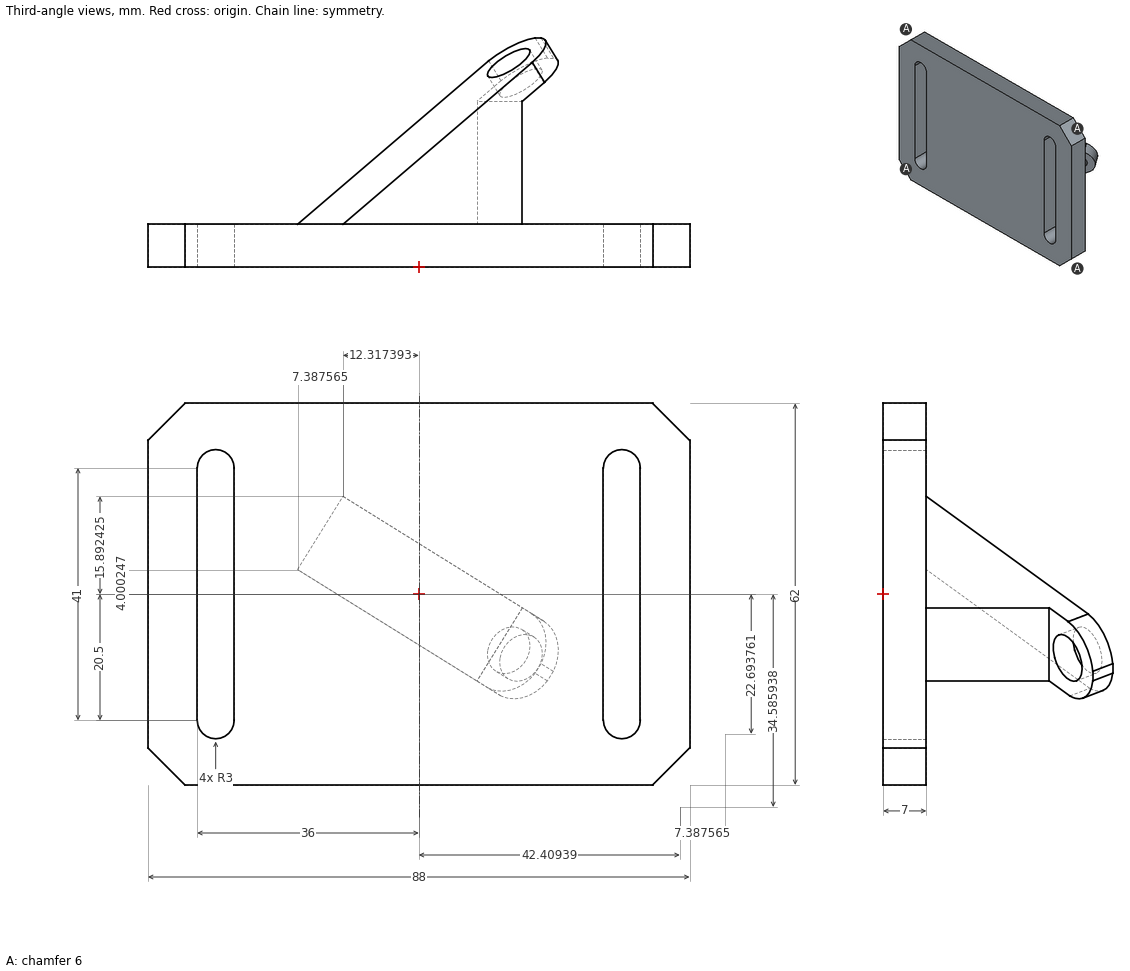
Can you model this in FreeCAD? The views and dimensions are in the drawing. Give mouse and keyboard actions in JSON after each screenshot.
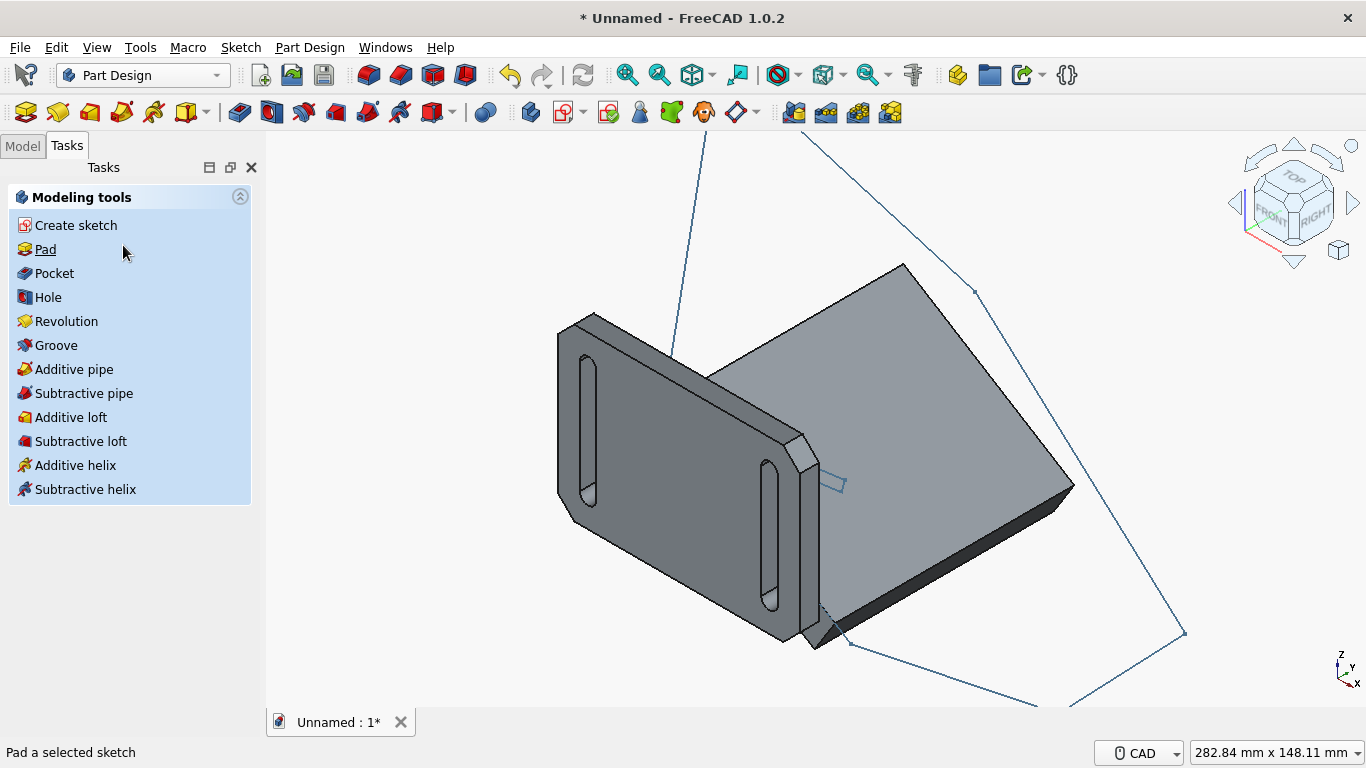
{"action": "left_click", "coordinate": [240, 112]}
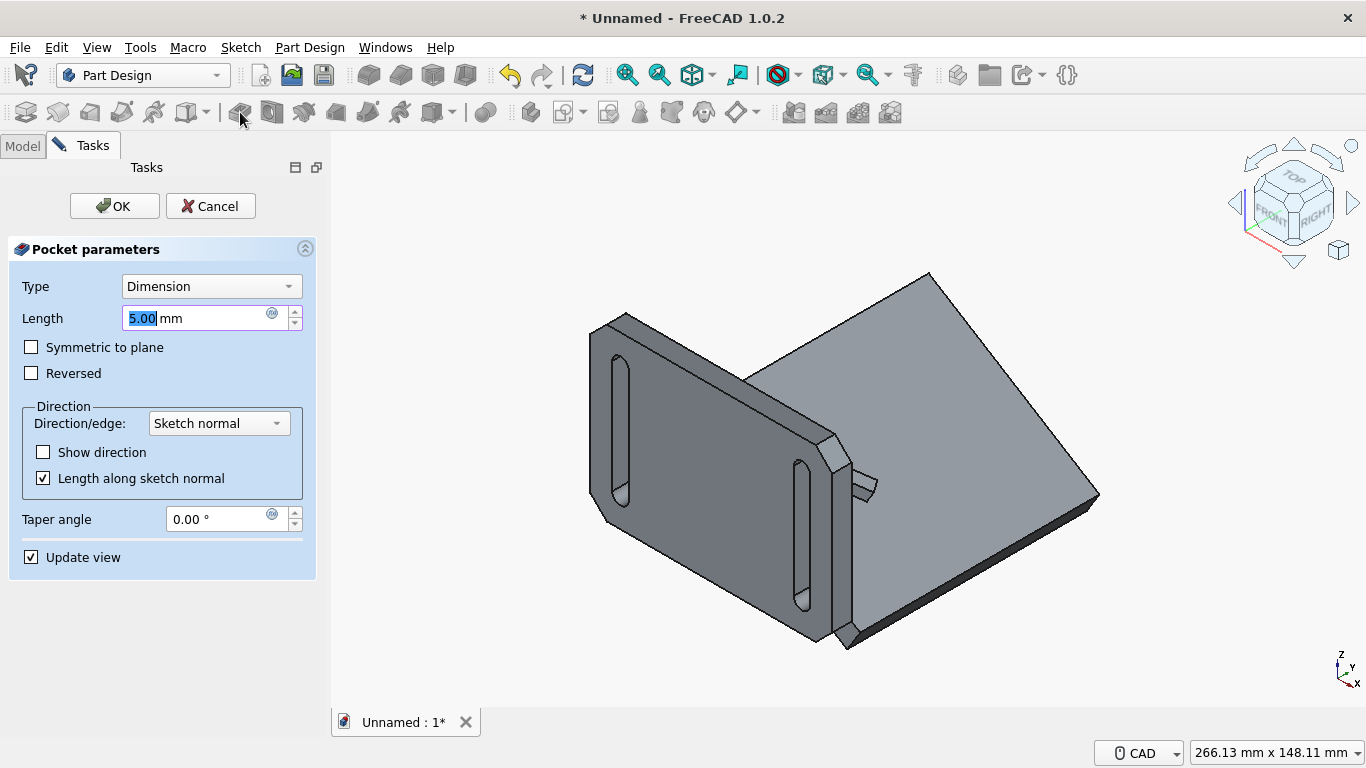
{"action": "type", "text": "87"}
{"action": "key", "text": "Tab"}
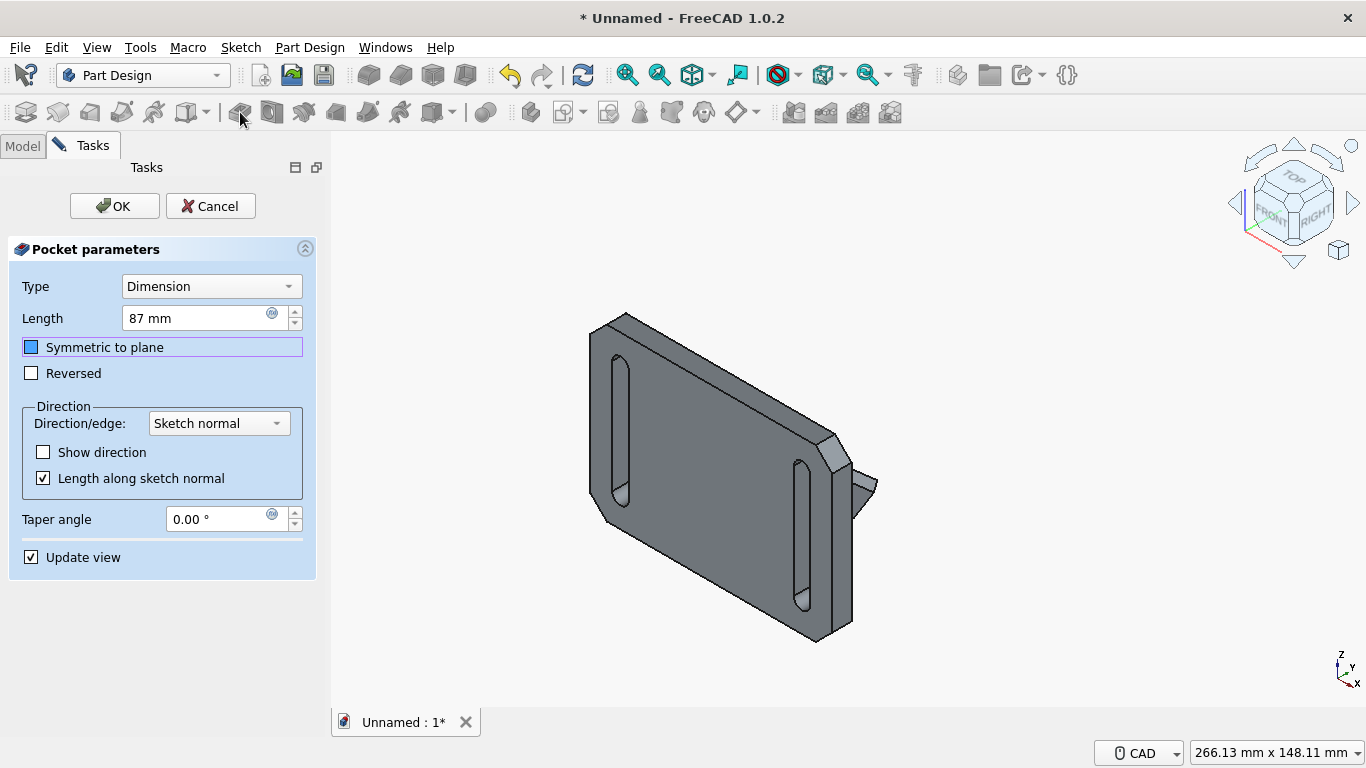
{"action": "left_click", "coordinate": [115, 206]}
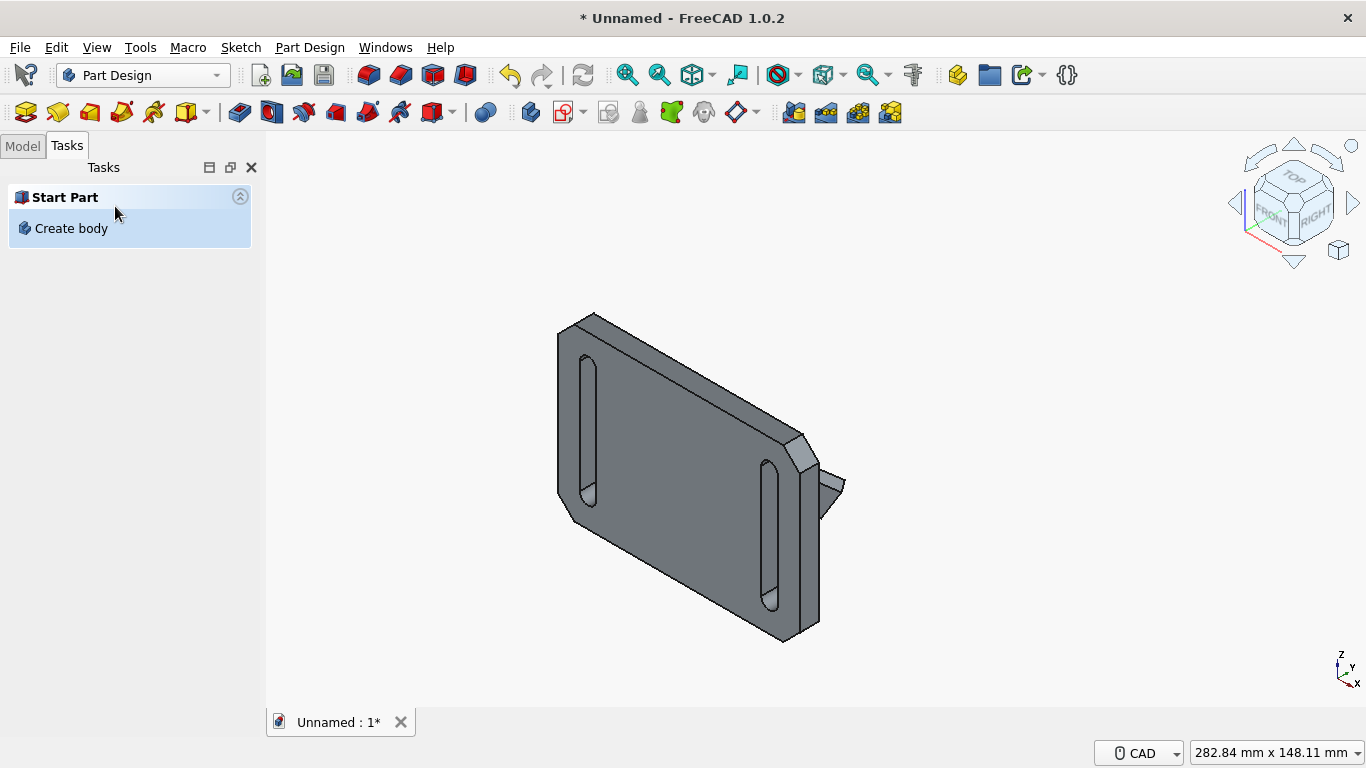
{"action": "key", "text": "4"}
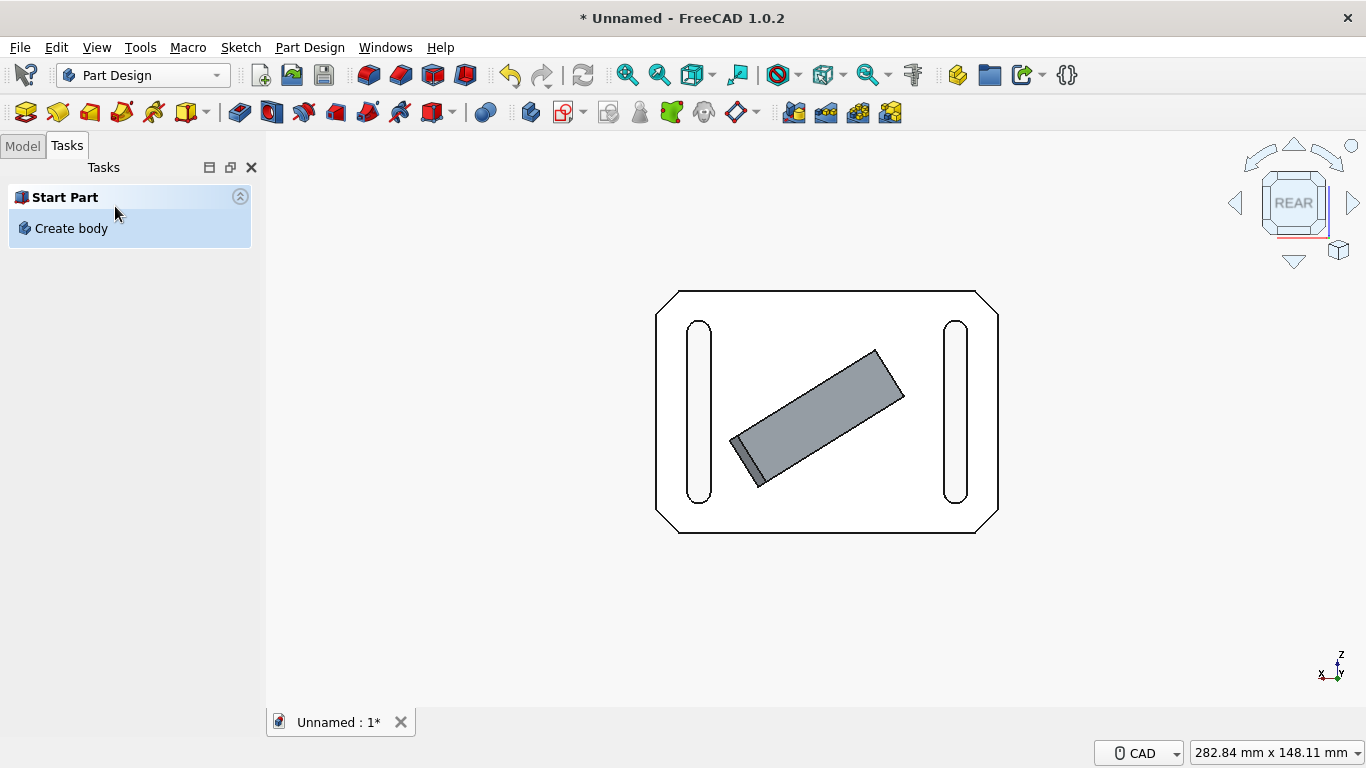
{"action": "left_click", "coordinate": [628, 76]}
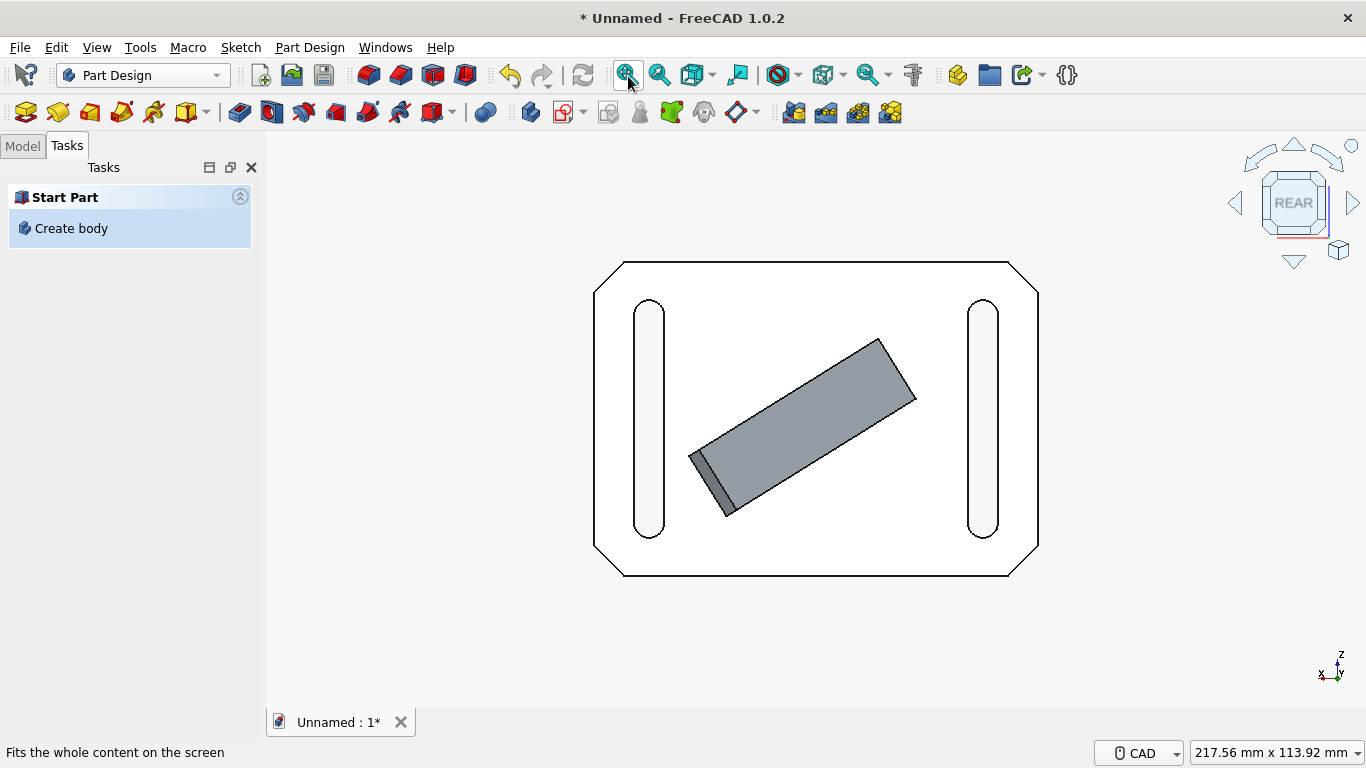
{"action": "left_click", "coordinate": [859, 392]}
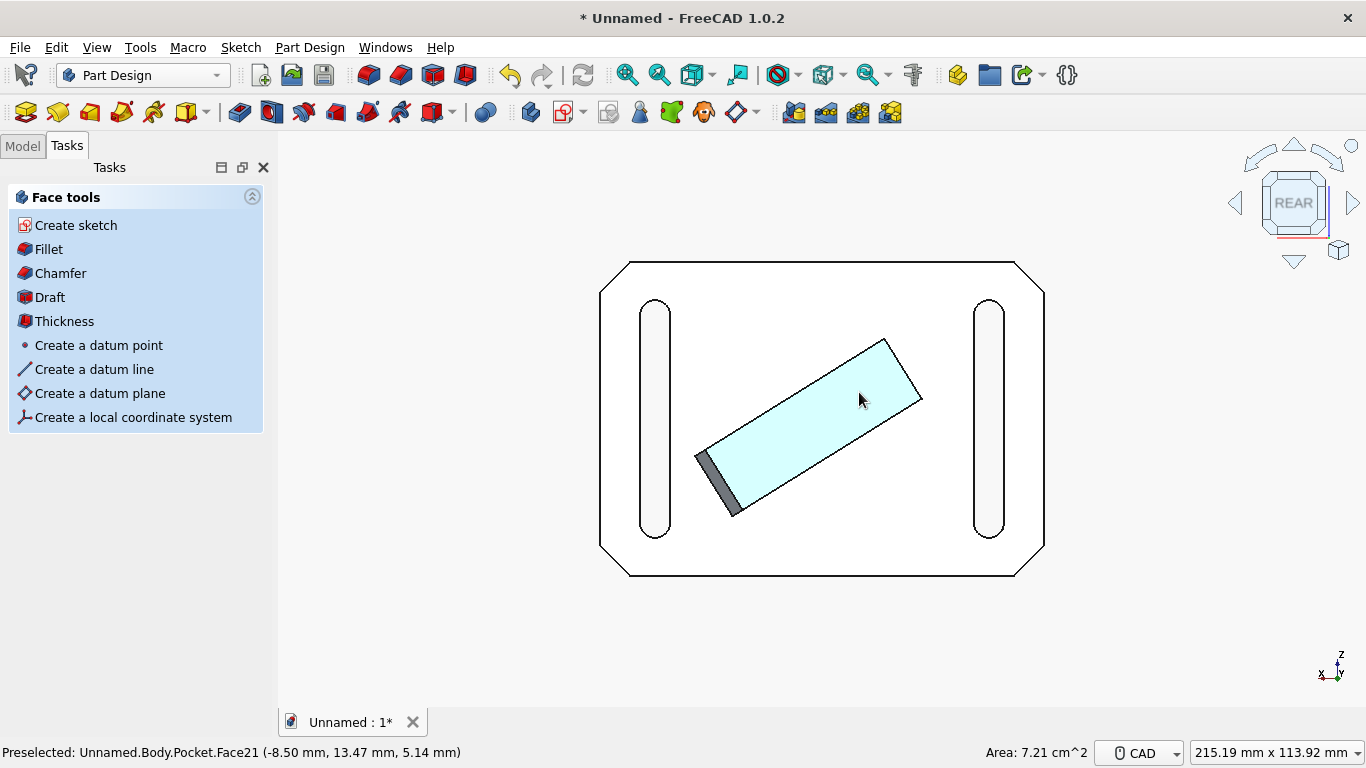
{"action": "left_click", "coordinate": [564, 112]}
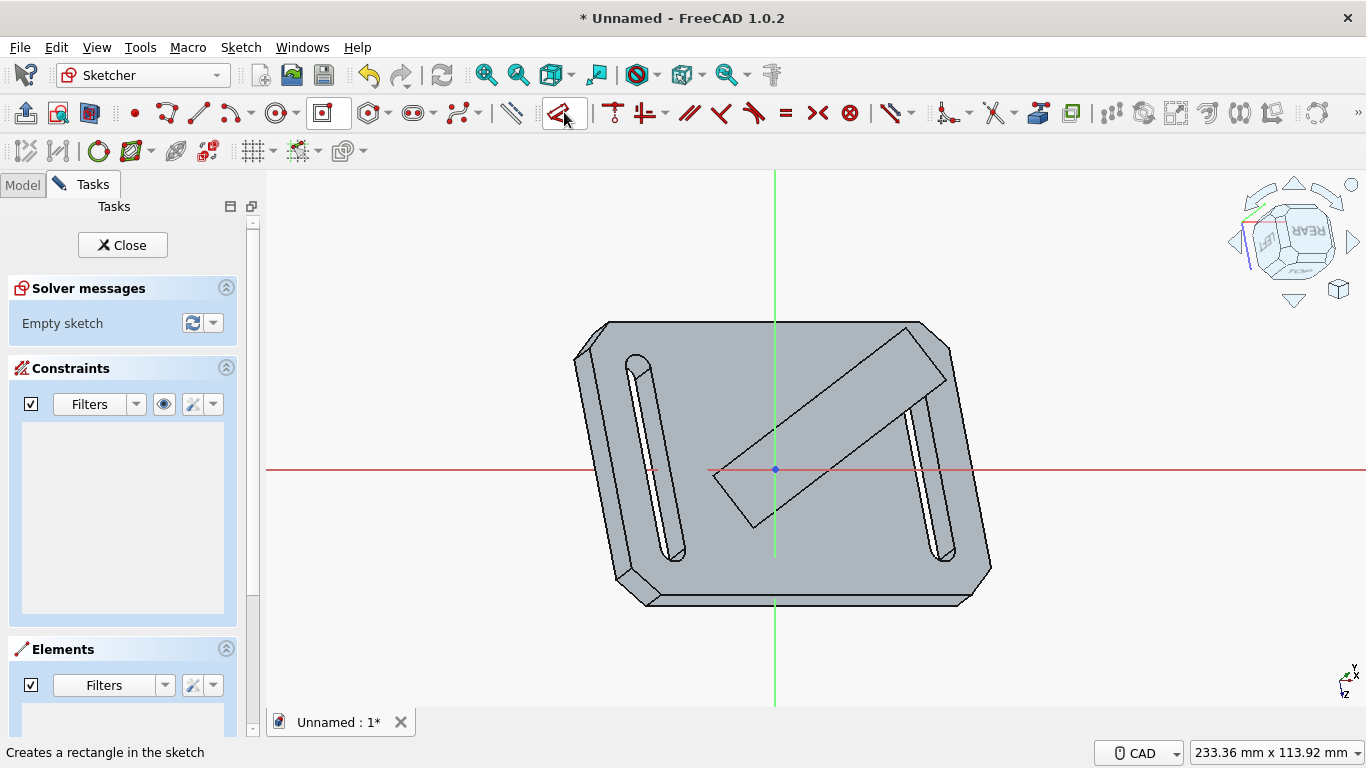
{"action": "left_click", "coordinate": [90, 114]}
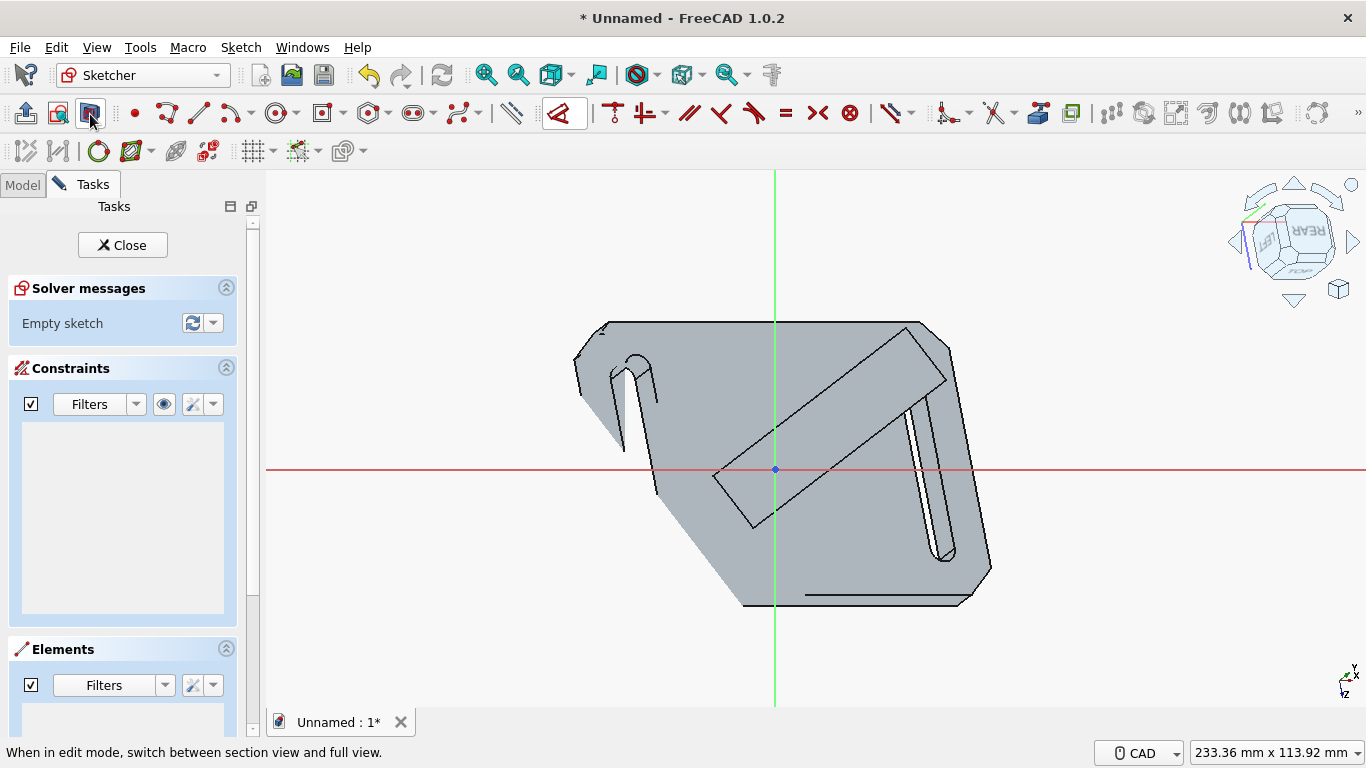
{"action": "scroll", "coordinate": [1043, 313], "scroll_direction": "up", "scroll_amount": 3}